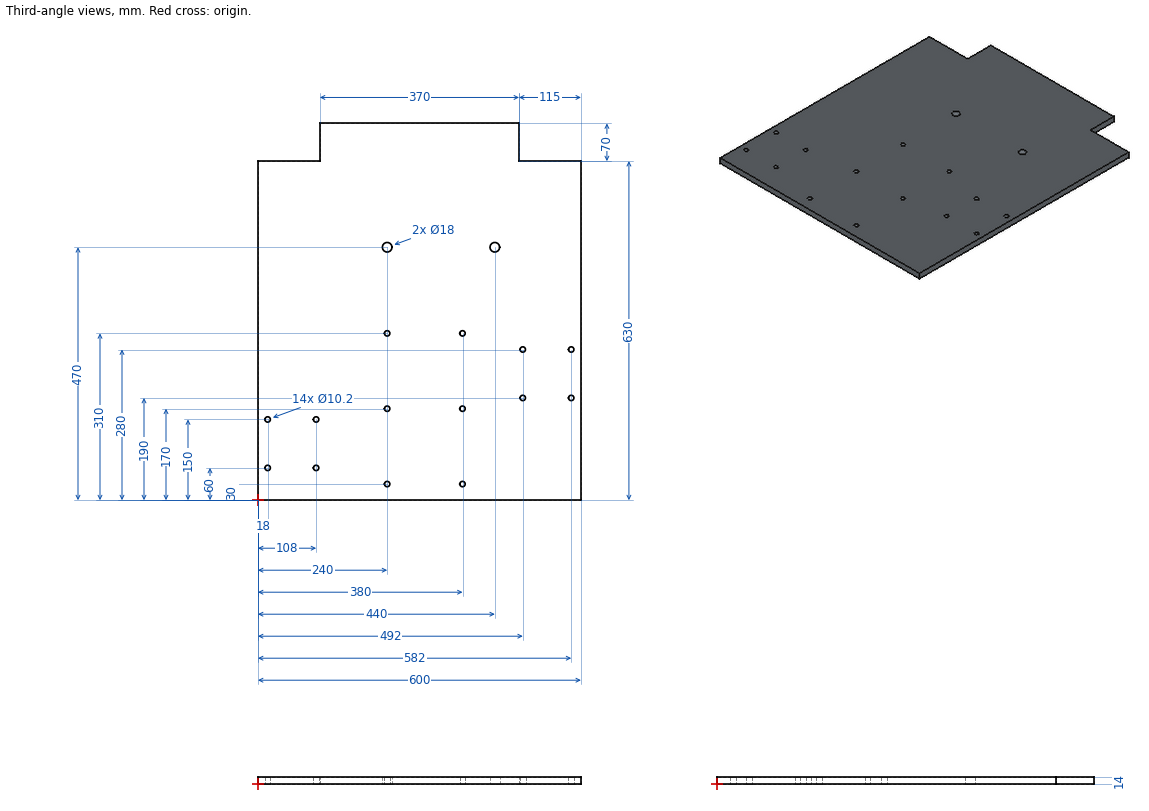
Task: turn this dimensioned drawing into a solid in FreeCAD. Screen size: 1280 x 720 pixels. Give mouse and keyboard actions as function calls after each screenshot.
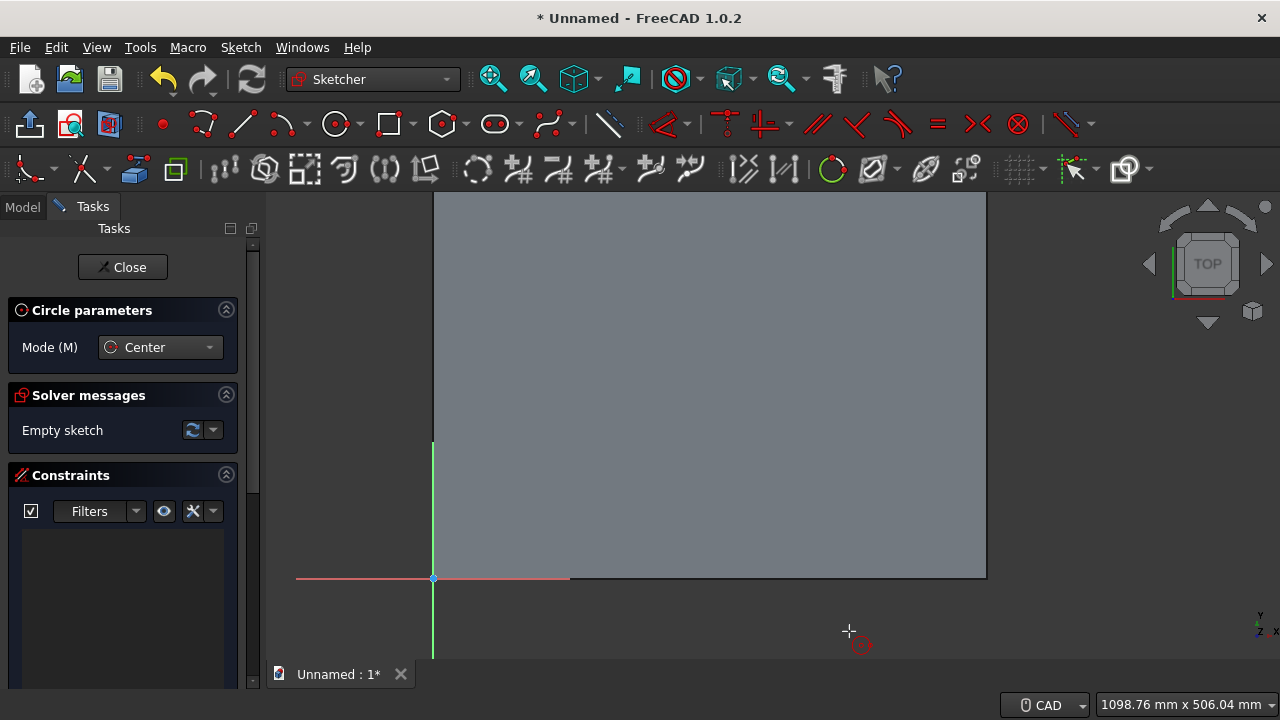
scroll(450, 440, up, 8)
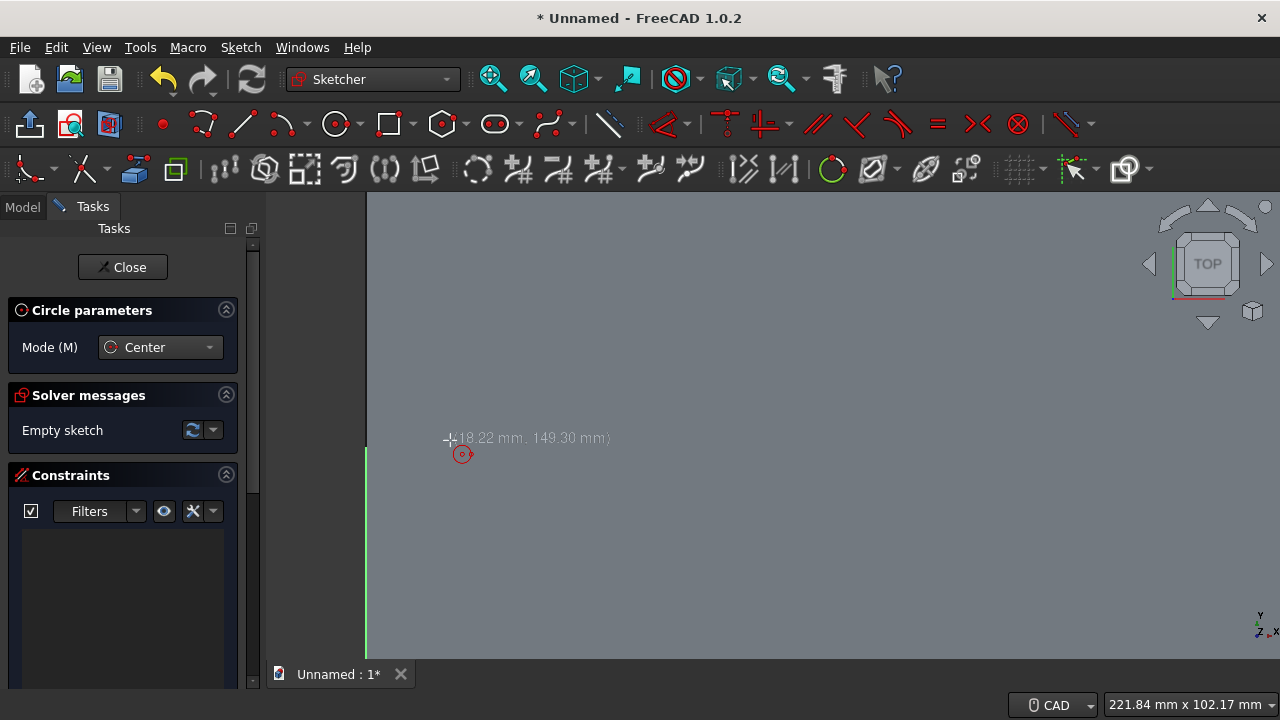
scroll(451, 431, down, 8)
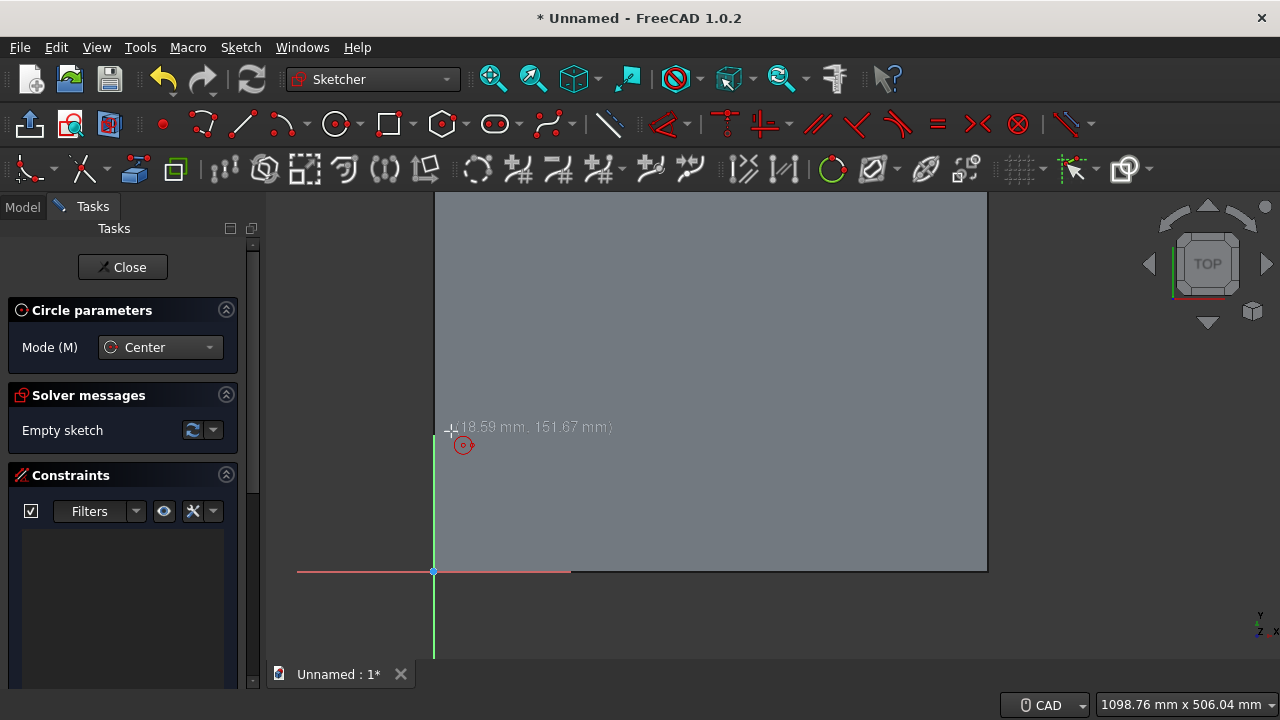
click(451, 433)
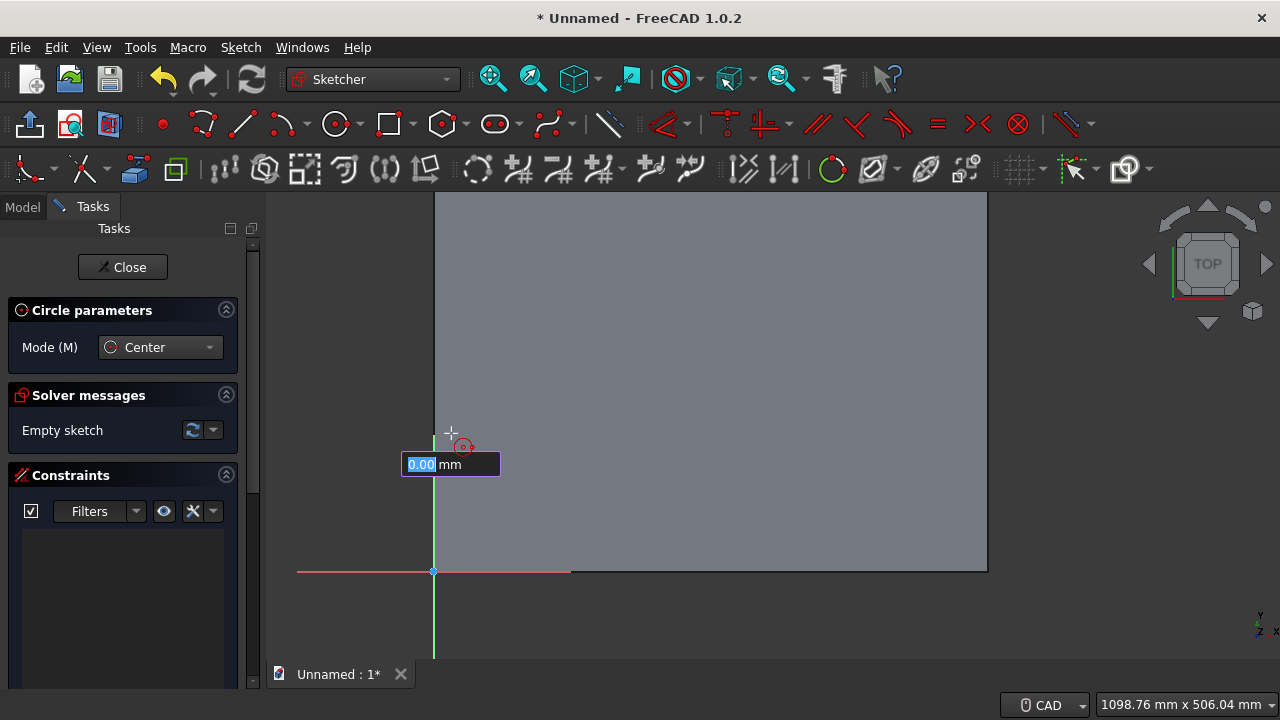
scroll(454, 430, up, 7)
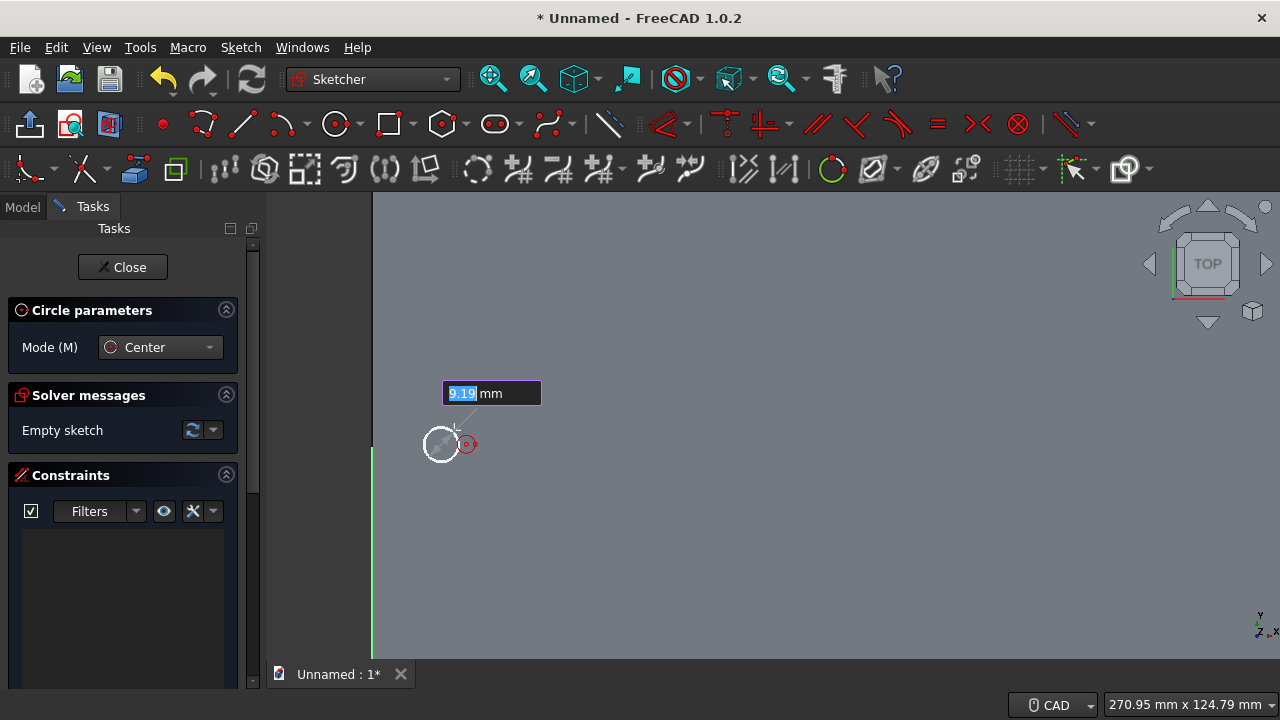
click(453, 428)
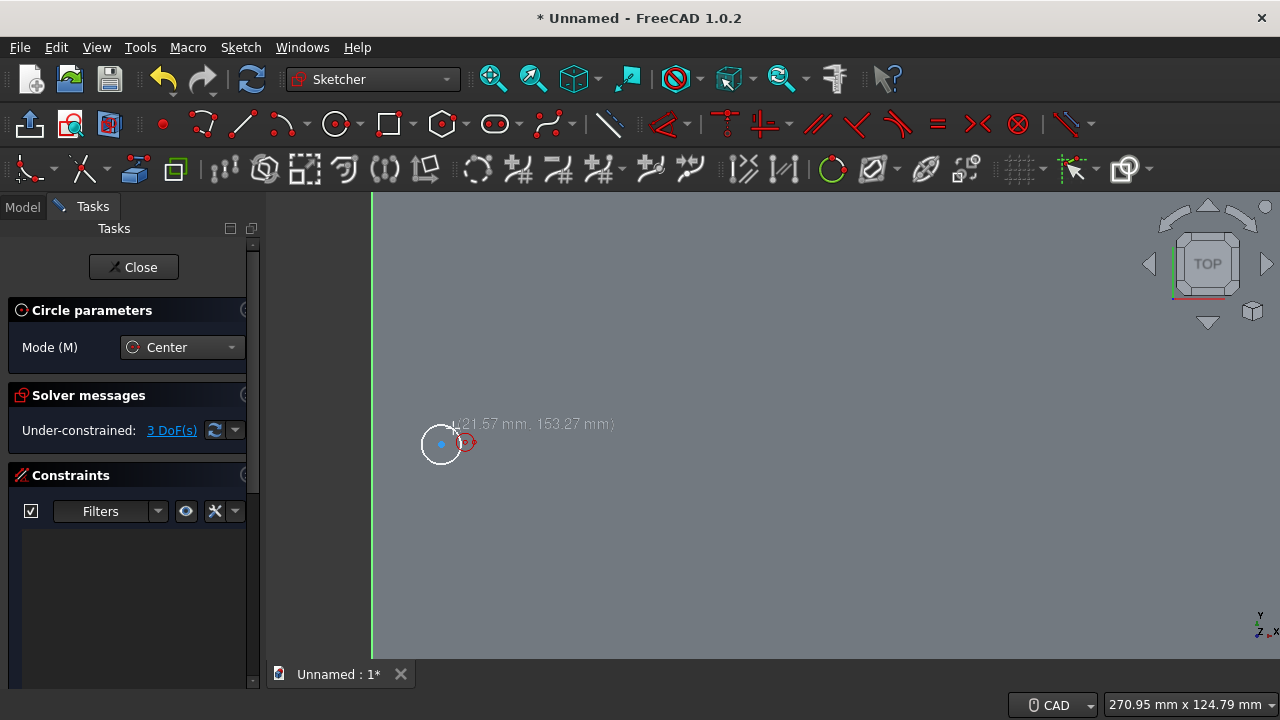
scroll(454, 430, down, 7)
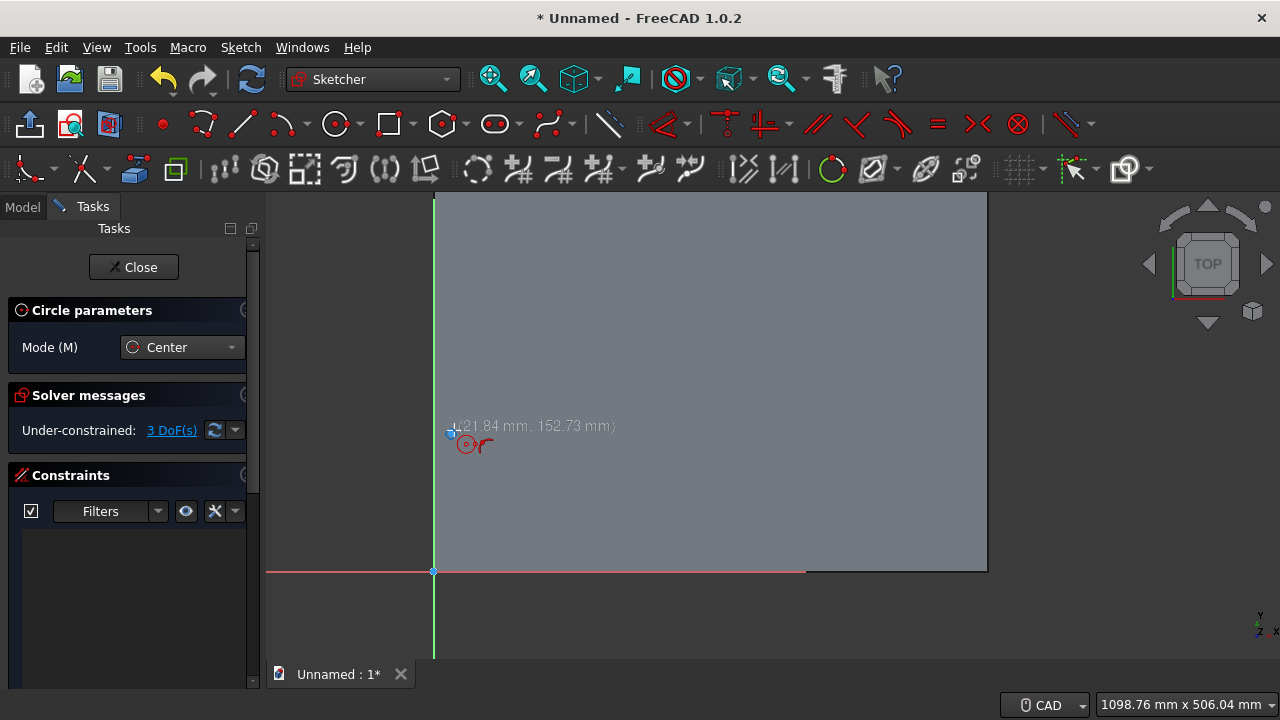
click(534, 433)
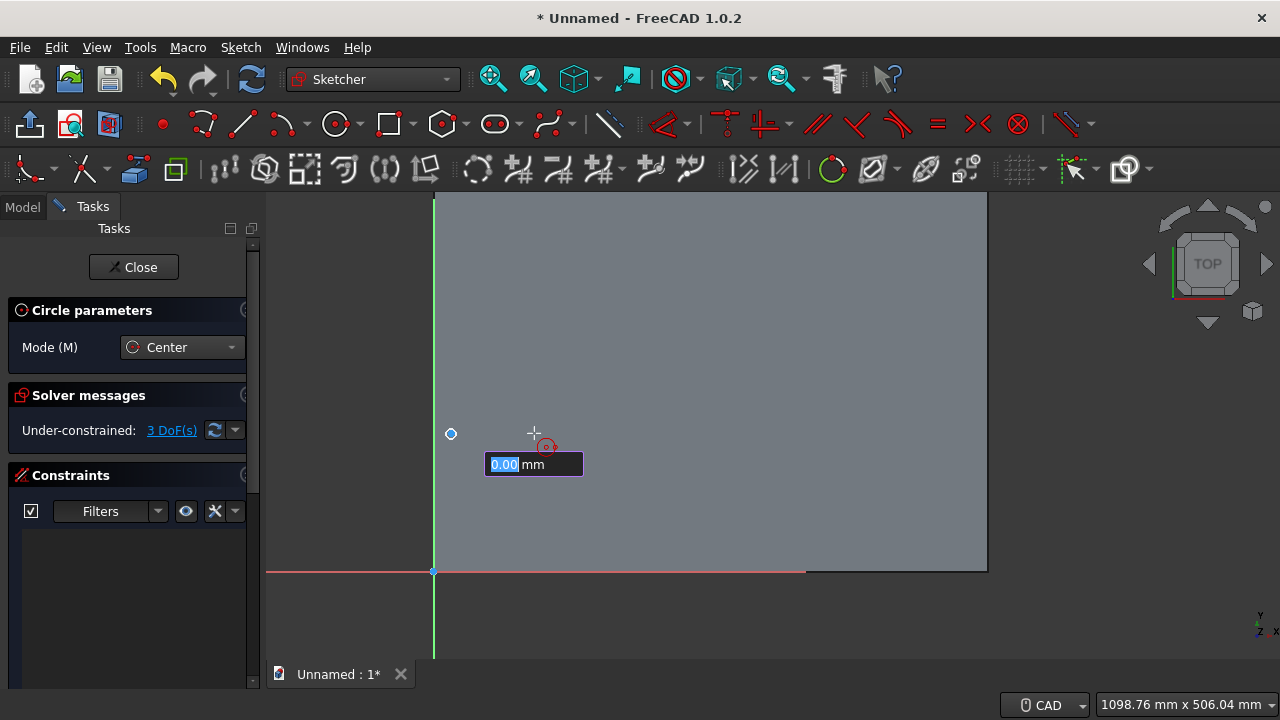
scroll(537, 430, up, 7)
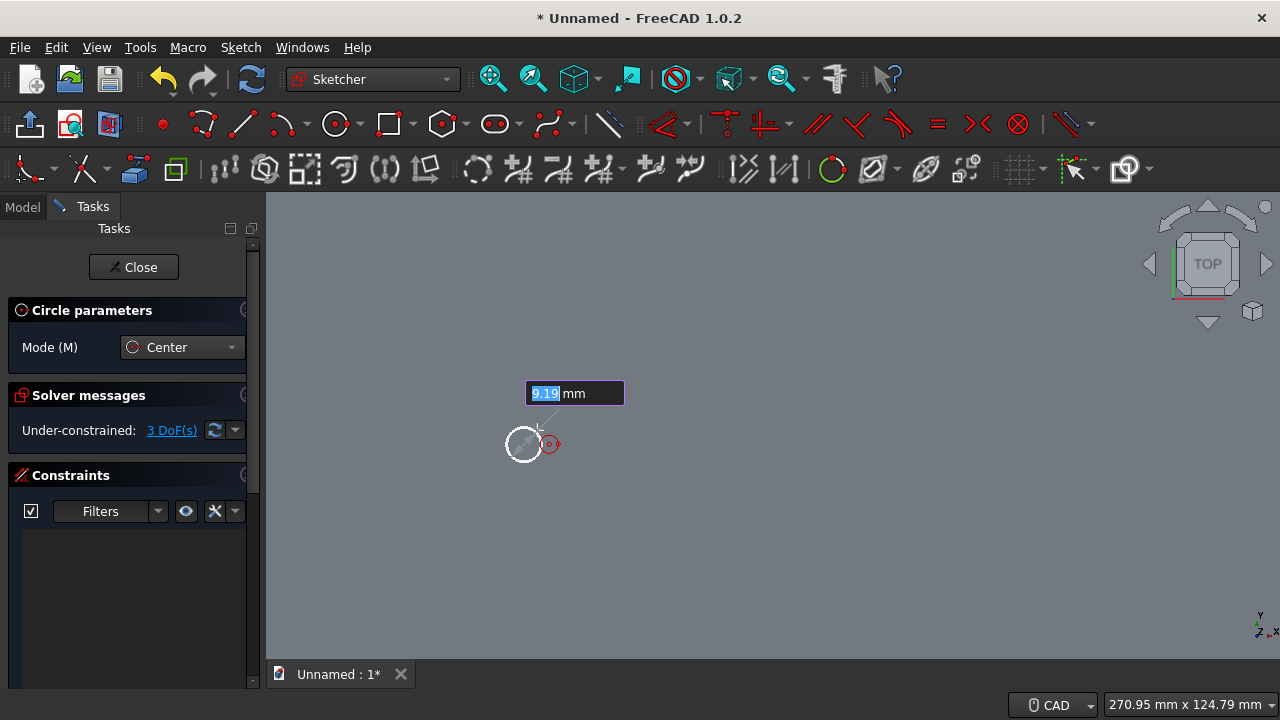
click(536, 428)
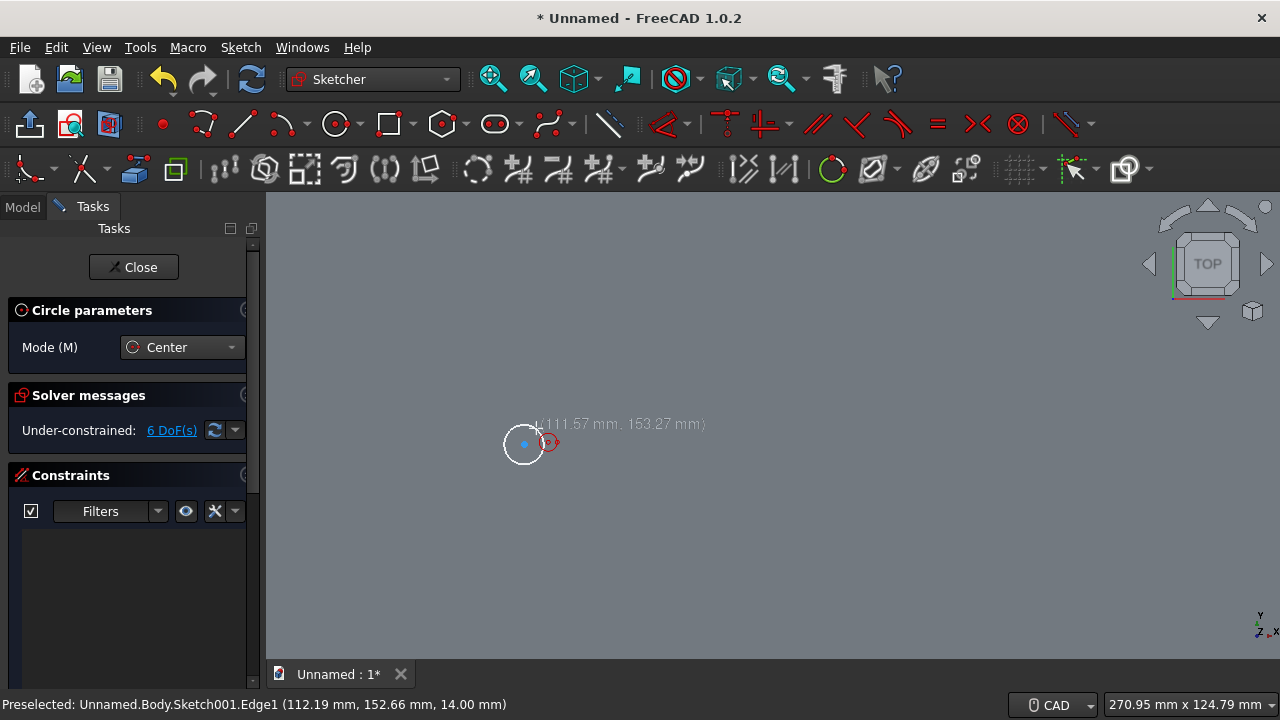
scroll(537, 430, down, 7)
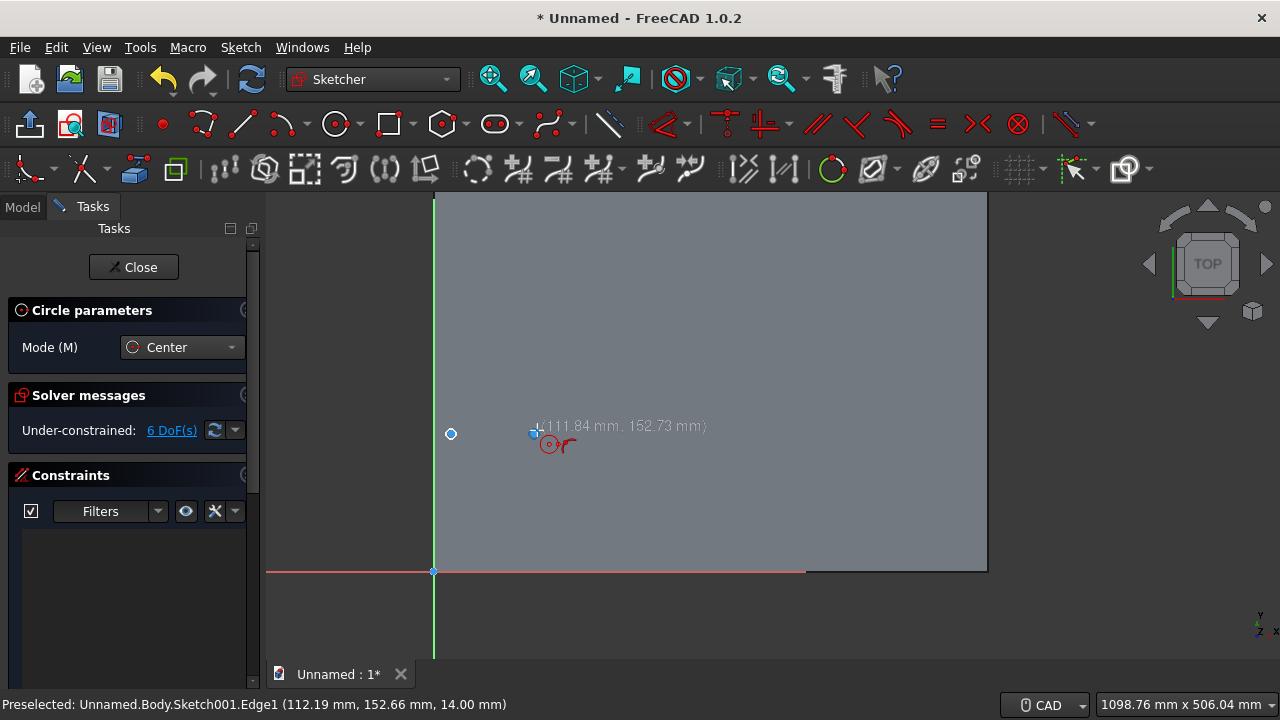
scroll(451, 516, up, 8)